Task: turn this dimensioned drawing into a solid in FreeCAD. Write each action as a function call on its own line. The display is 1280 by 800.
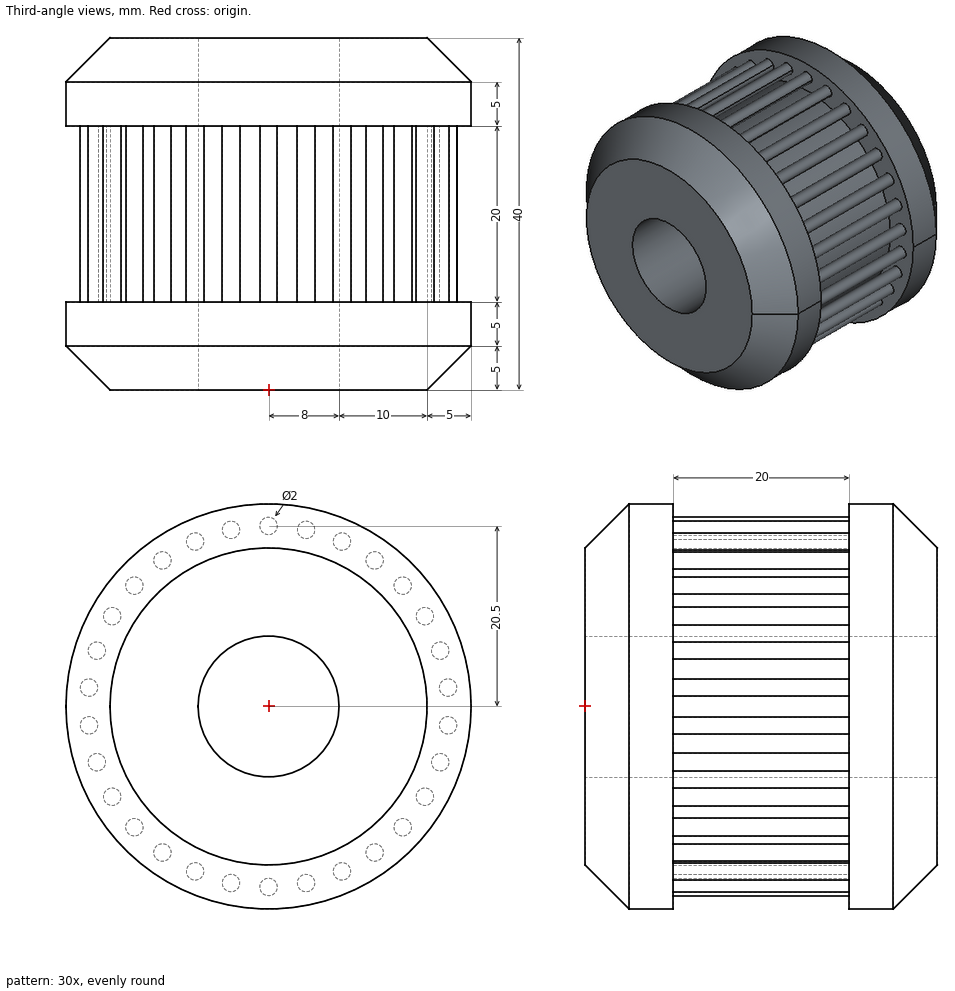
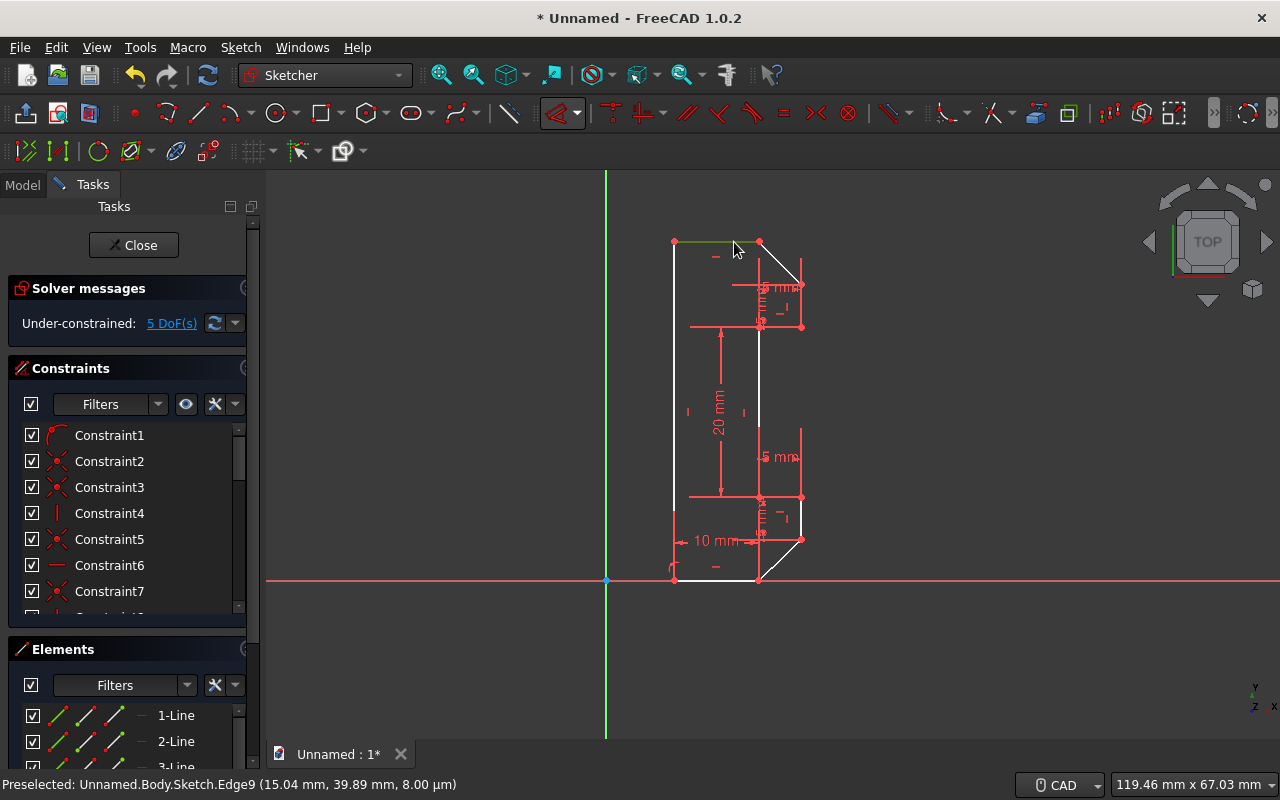
key(l)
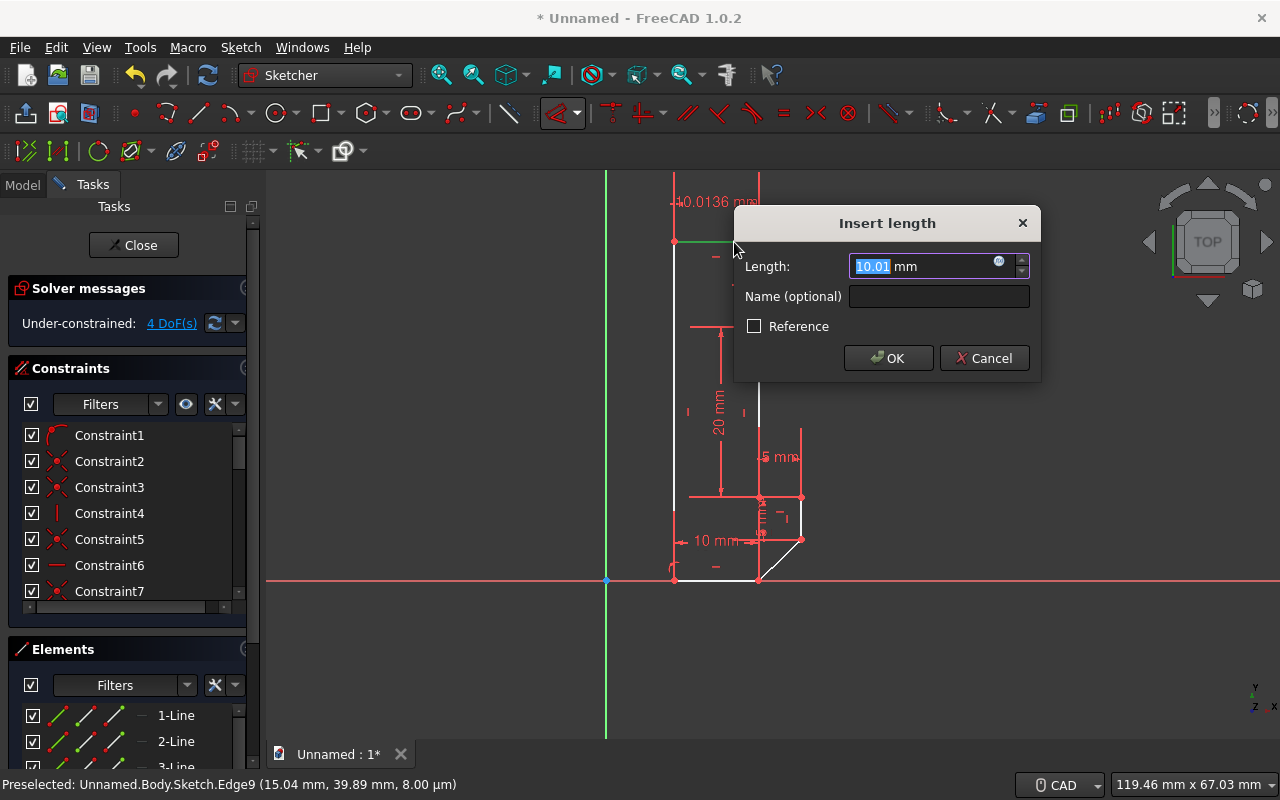
text(10)
key(Return)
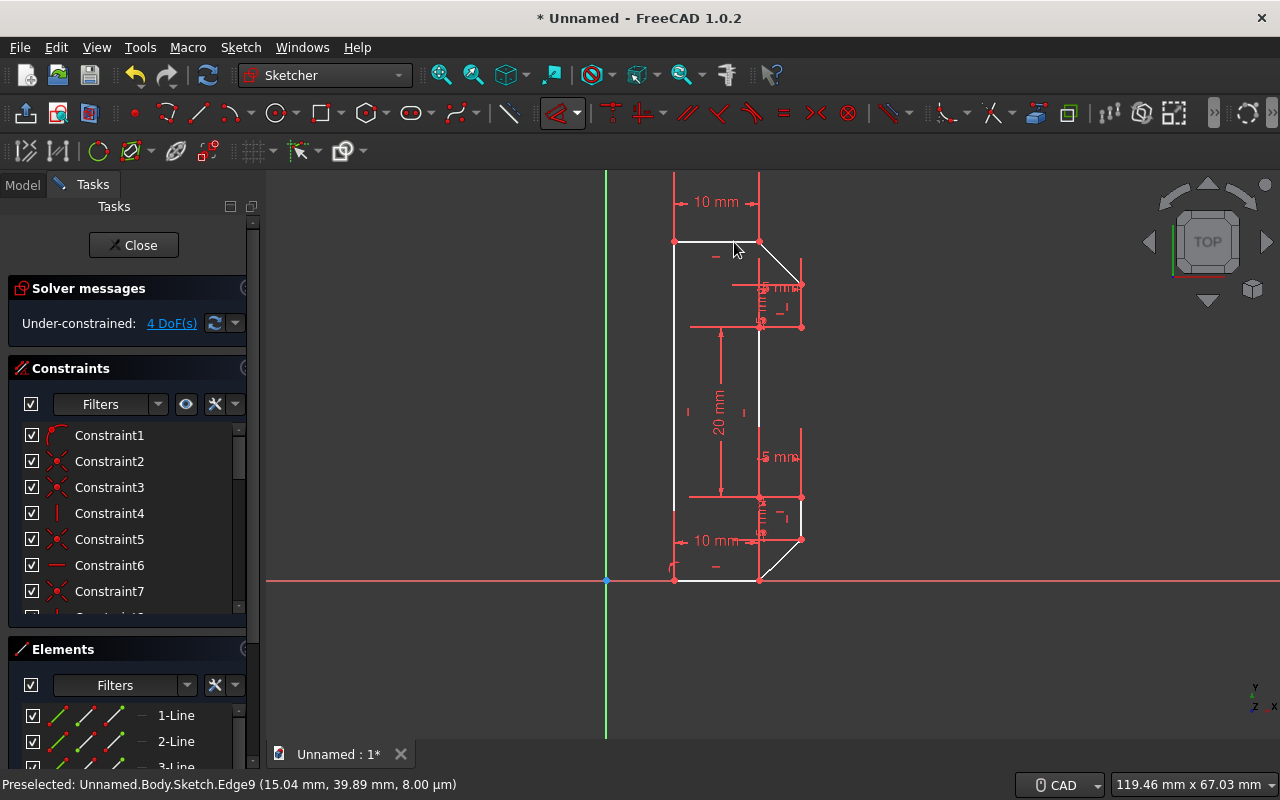
click(674, 344)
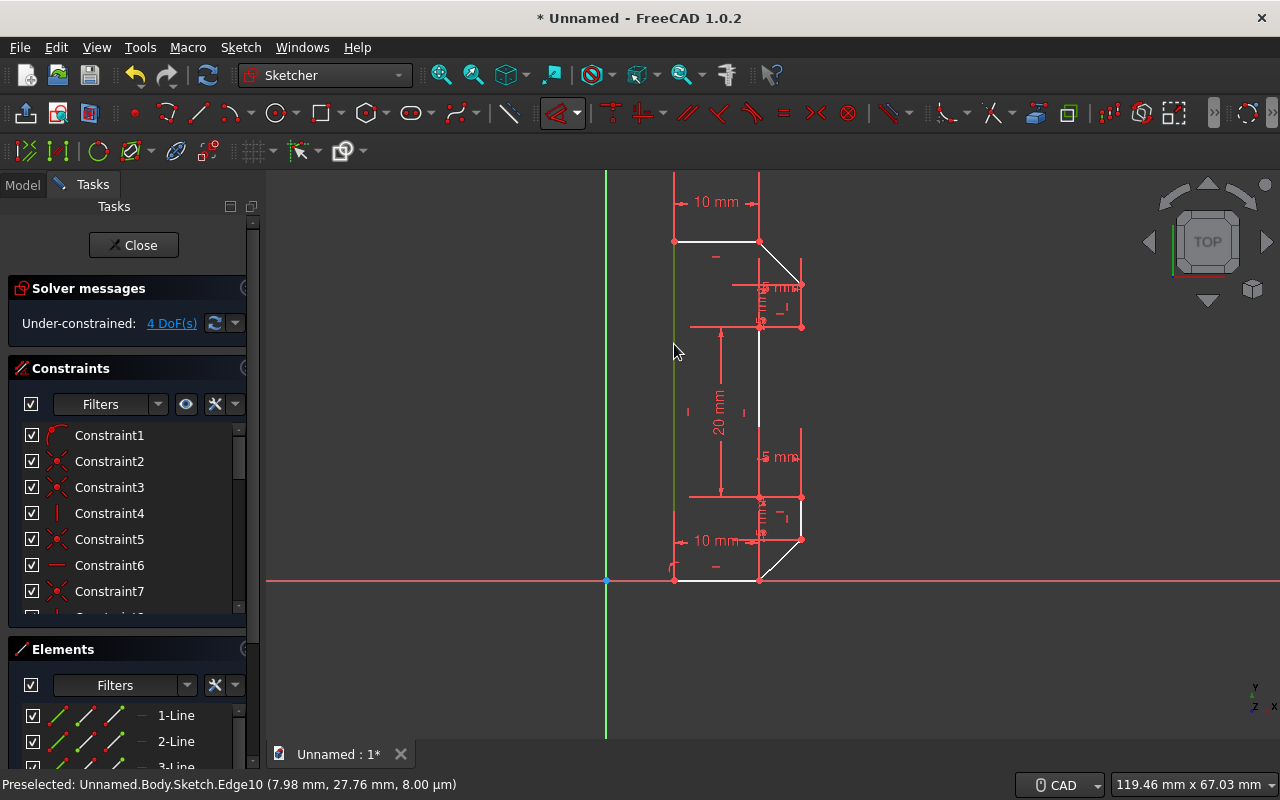
key(i)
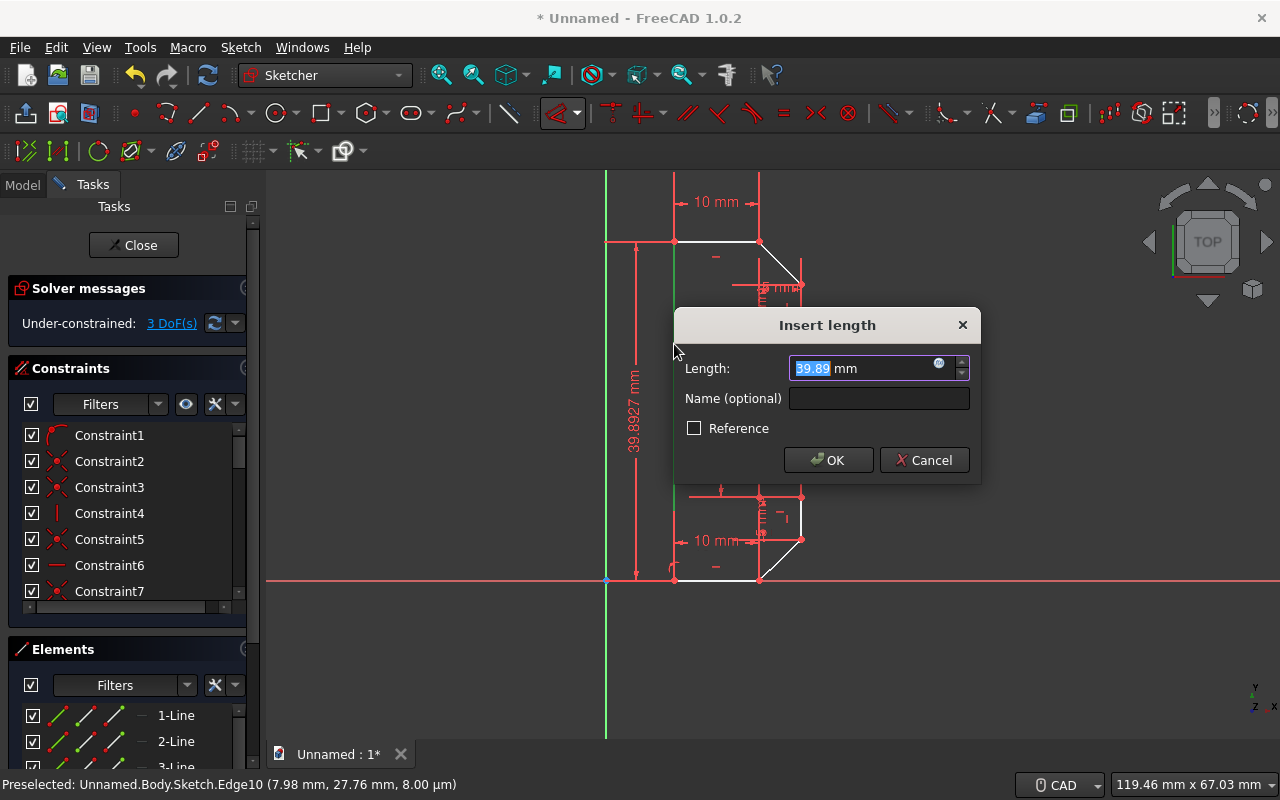
text(40)
key(Return)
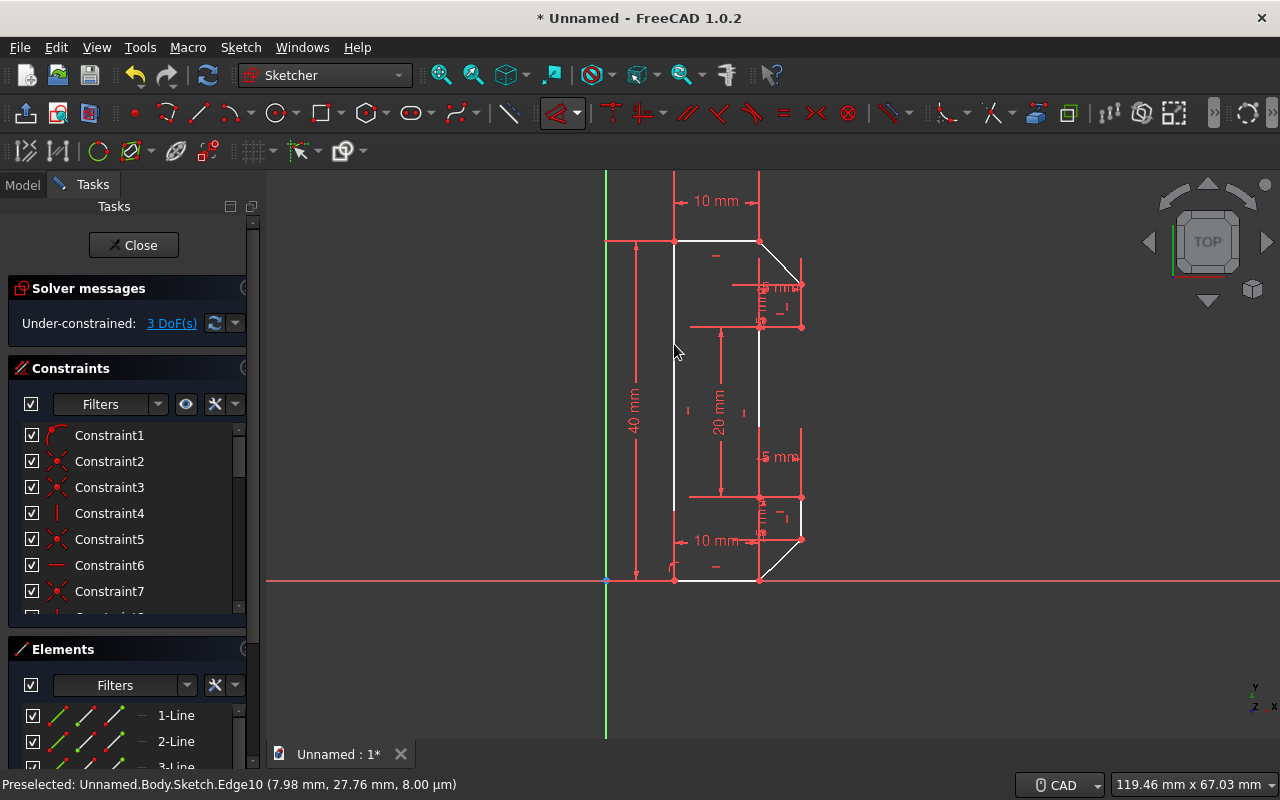
click(674, 581)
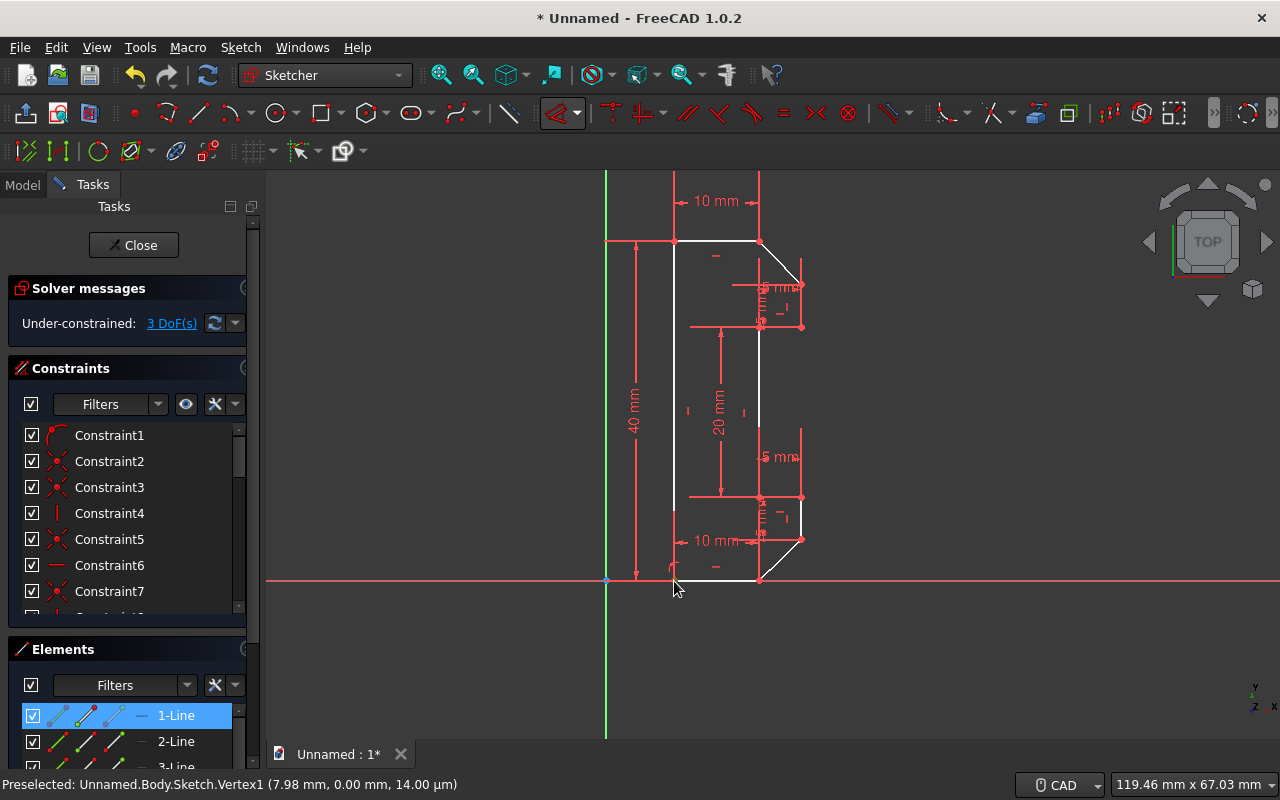
key(l)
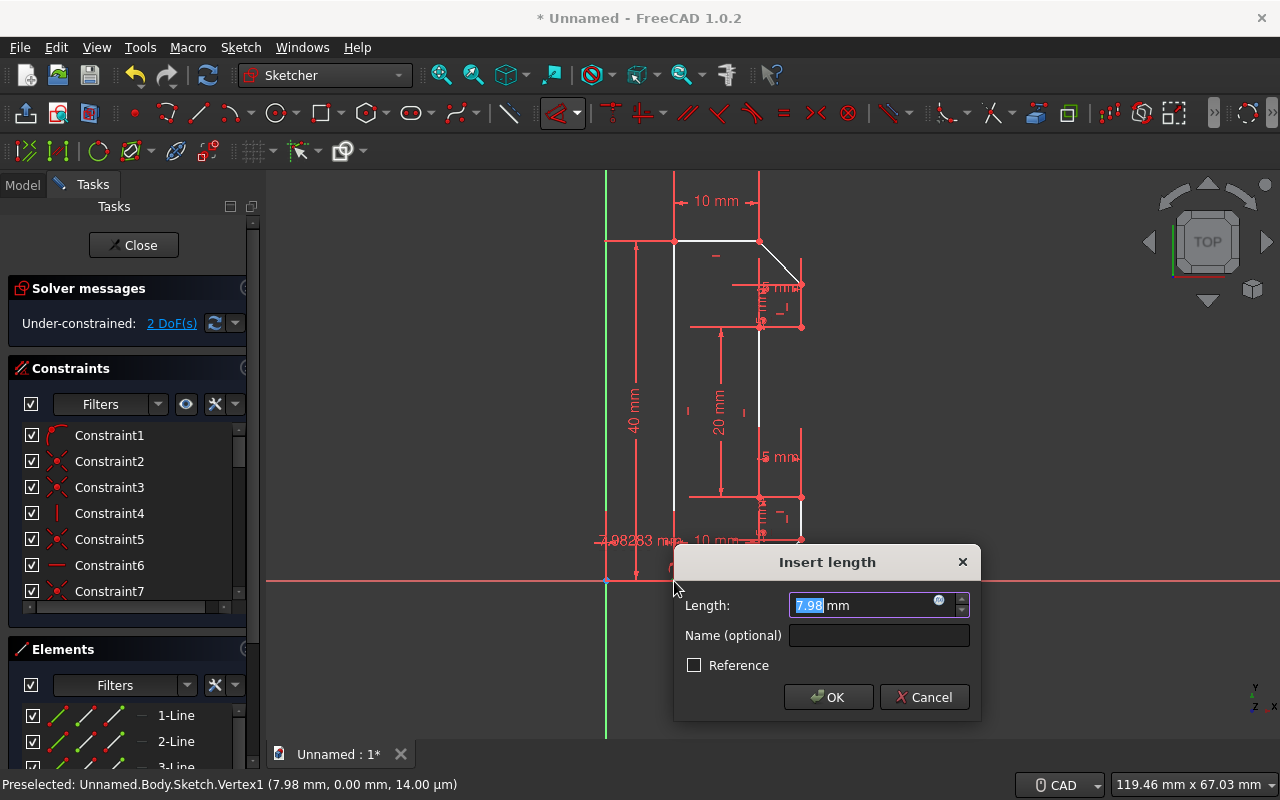
text(8)
key(Return)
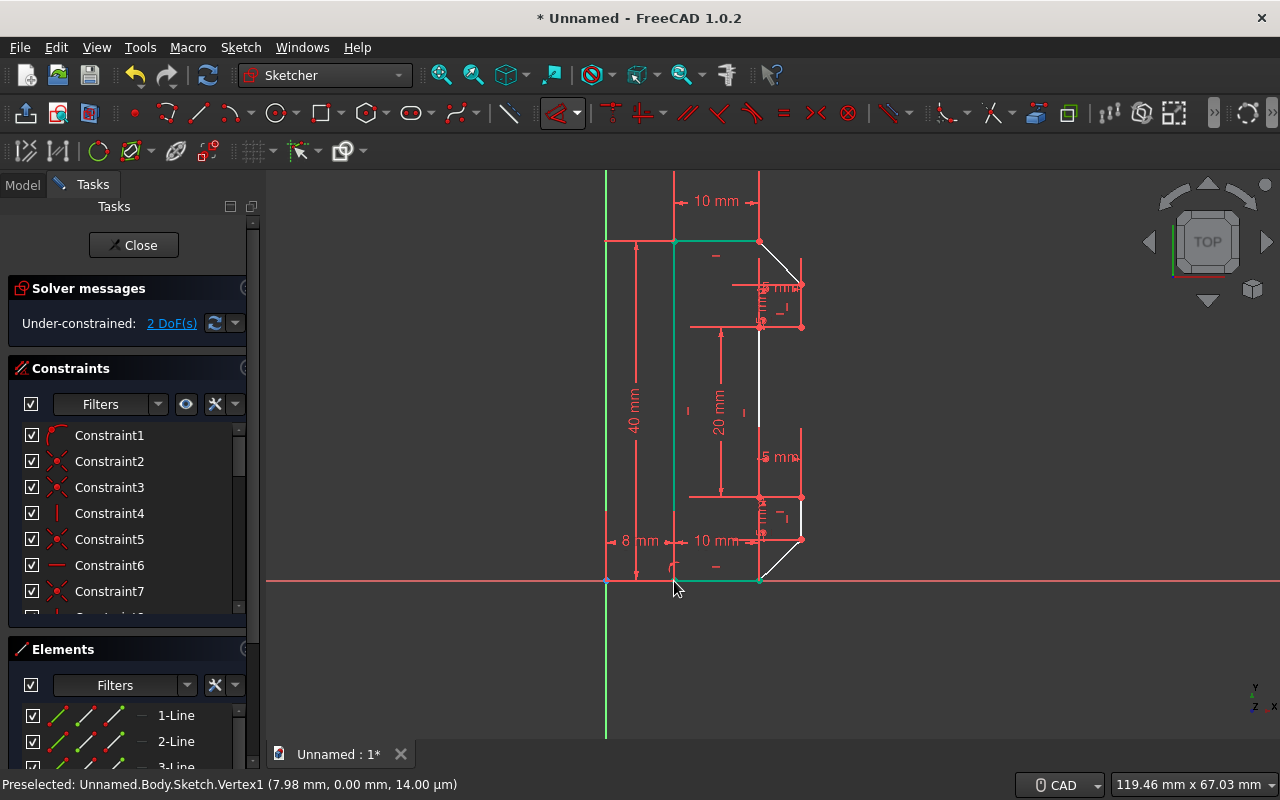
click(801, 540)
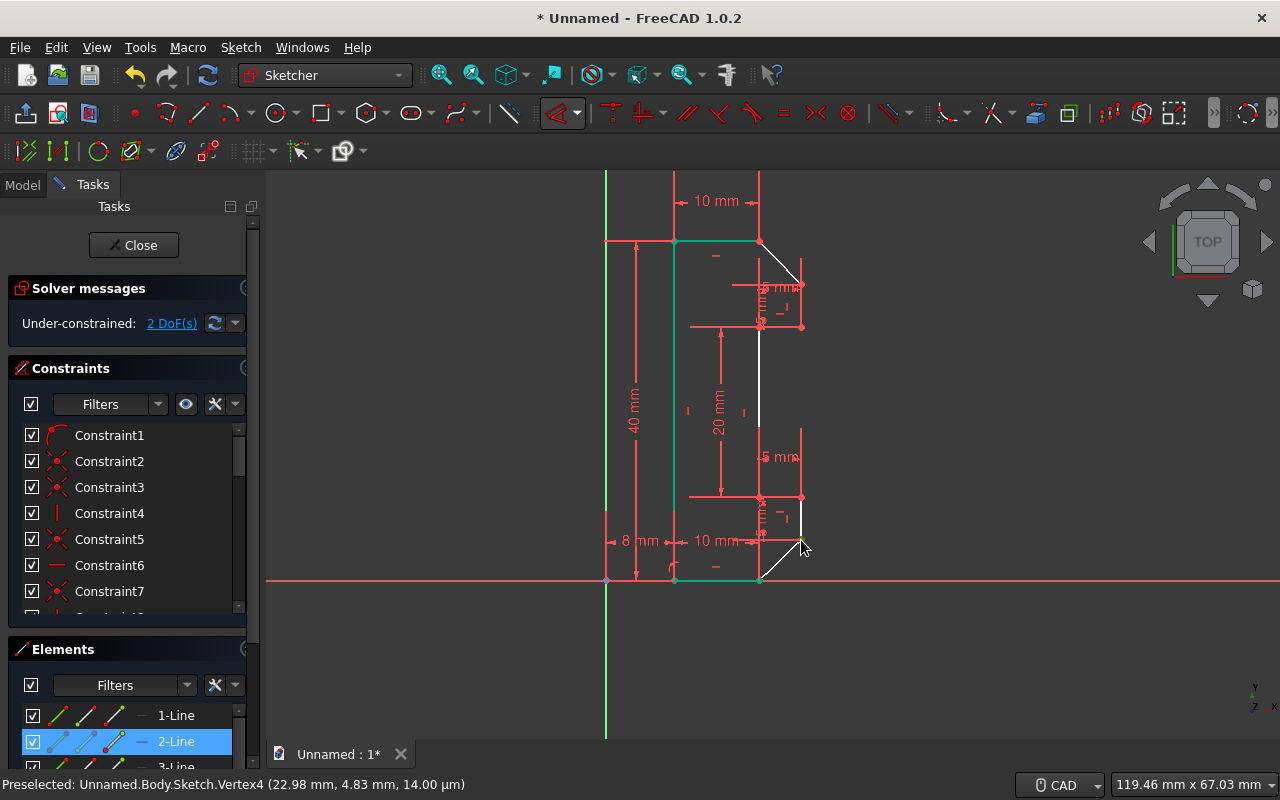
key(i)